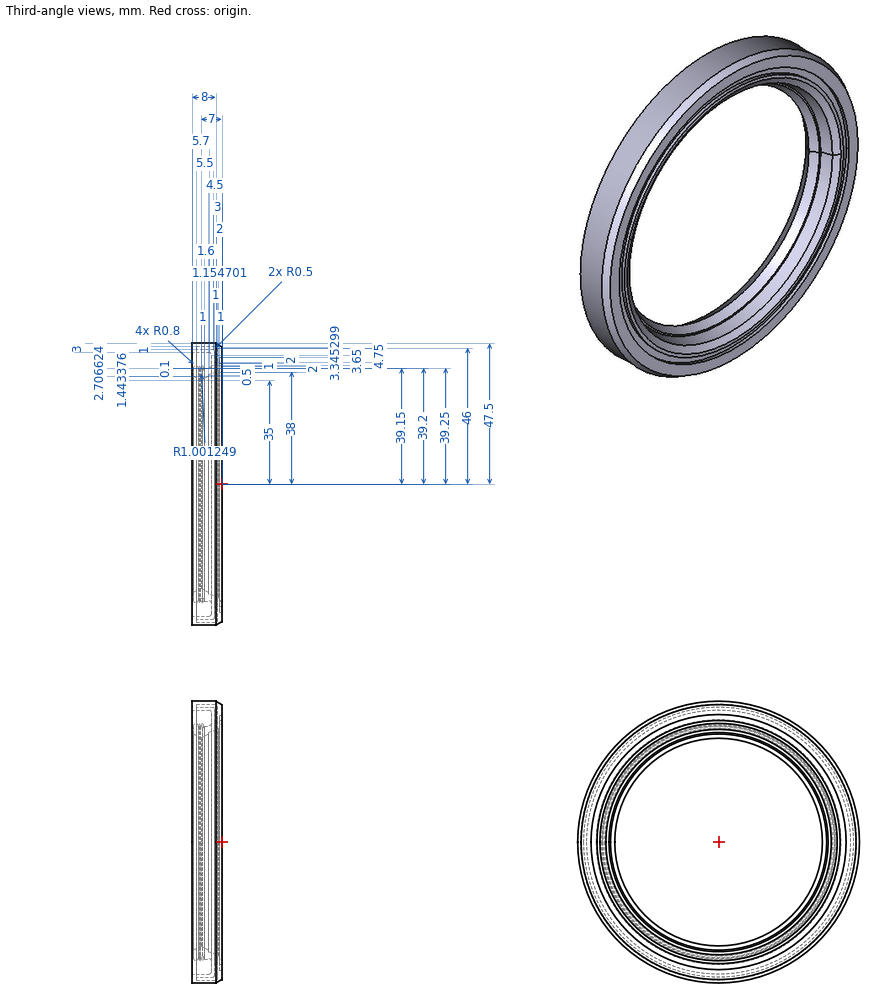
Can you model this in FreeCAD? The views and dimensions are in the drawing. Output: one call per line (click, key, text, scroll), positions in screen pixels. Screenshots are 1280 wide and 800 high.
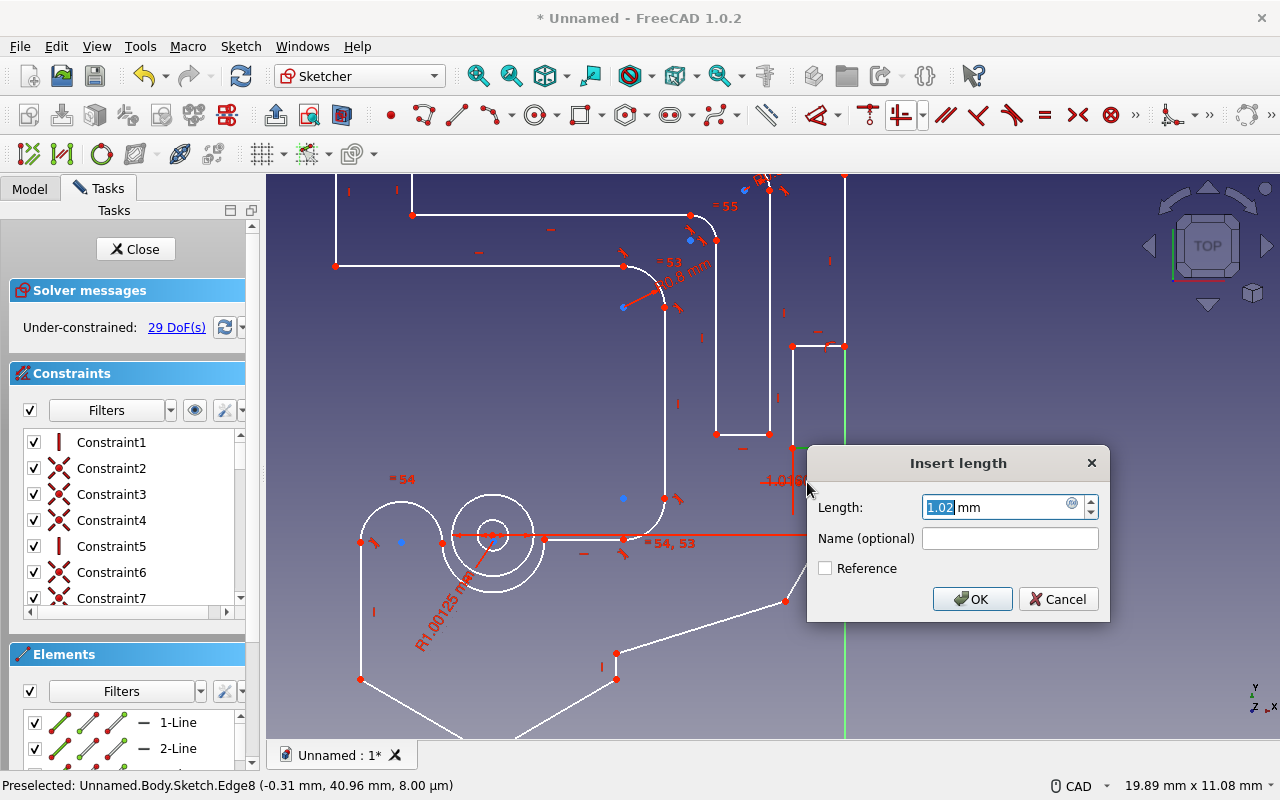
text(1)
key(Return)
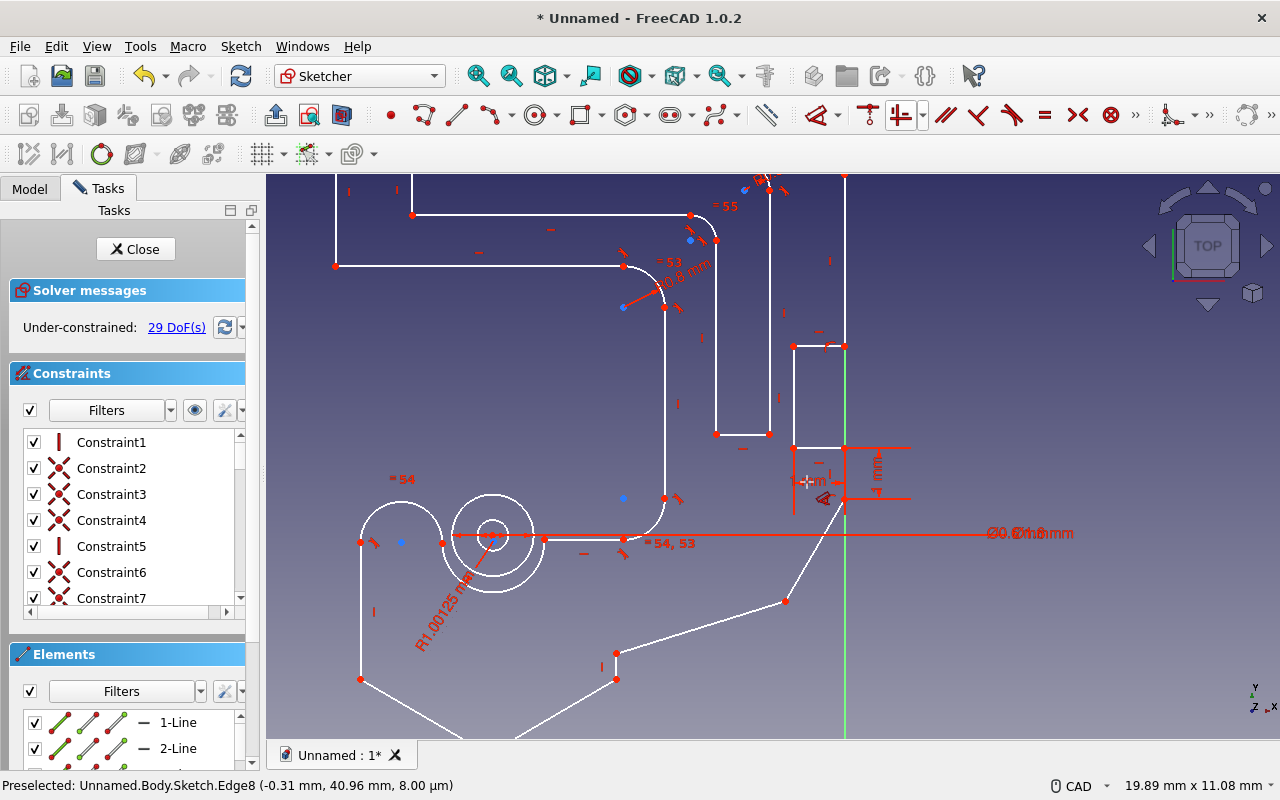
click(794, 417)
click(828, 397)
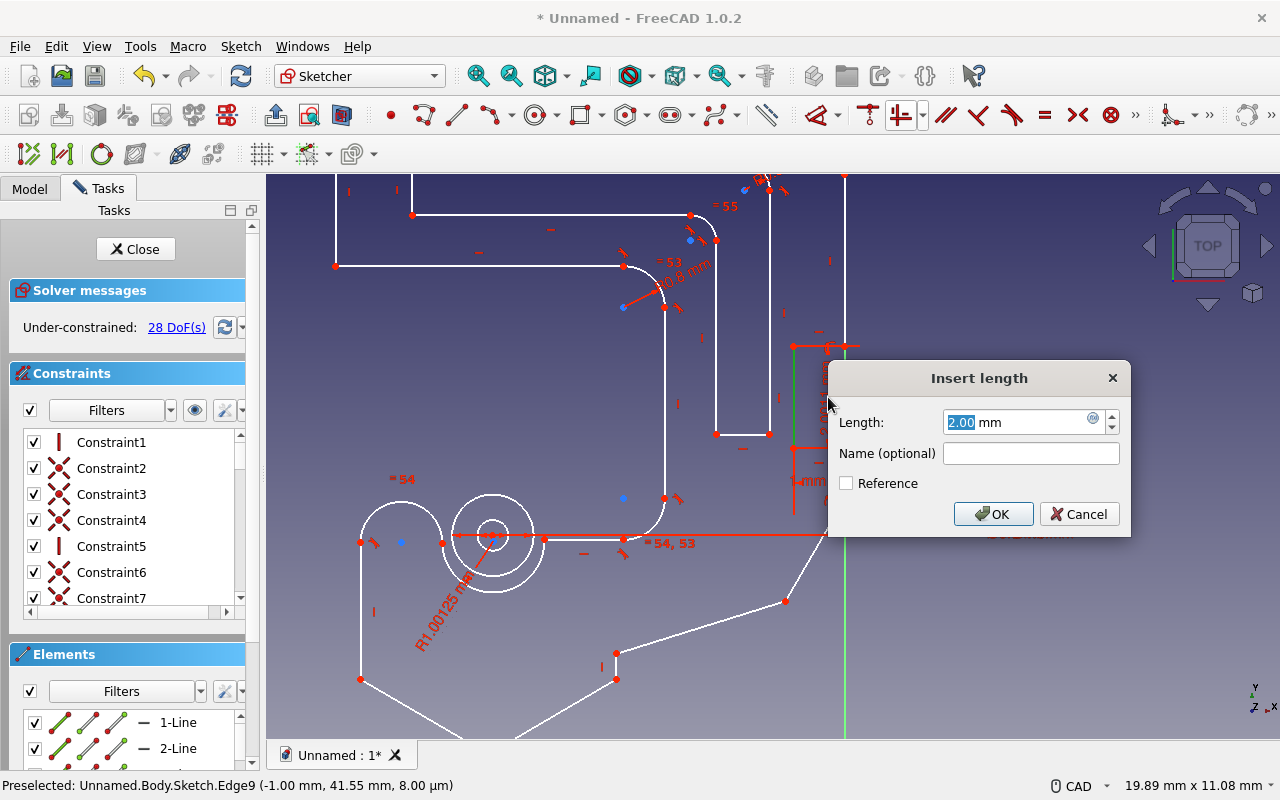
text(2)
key(Return)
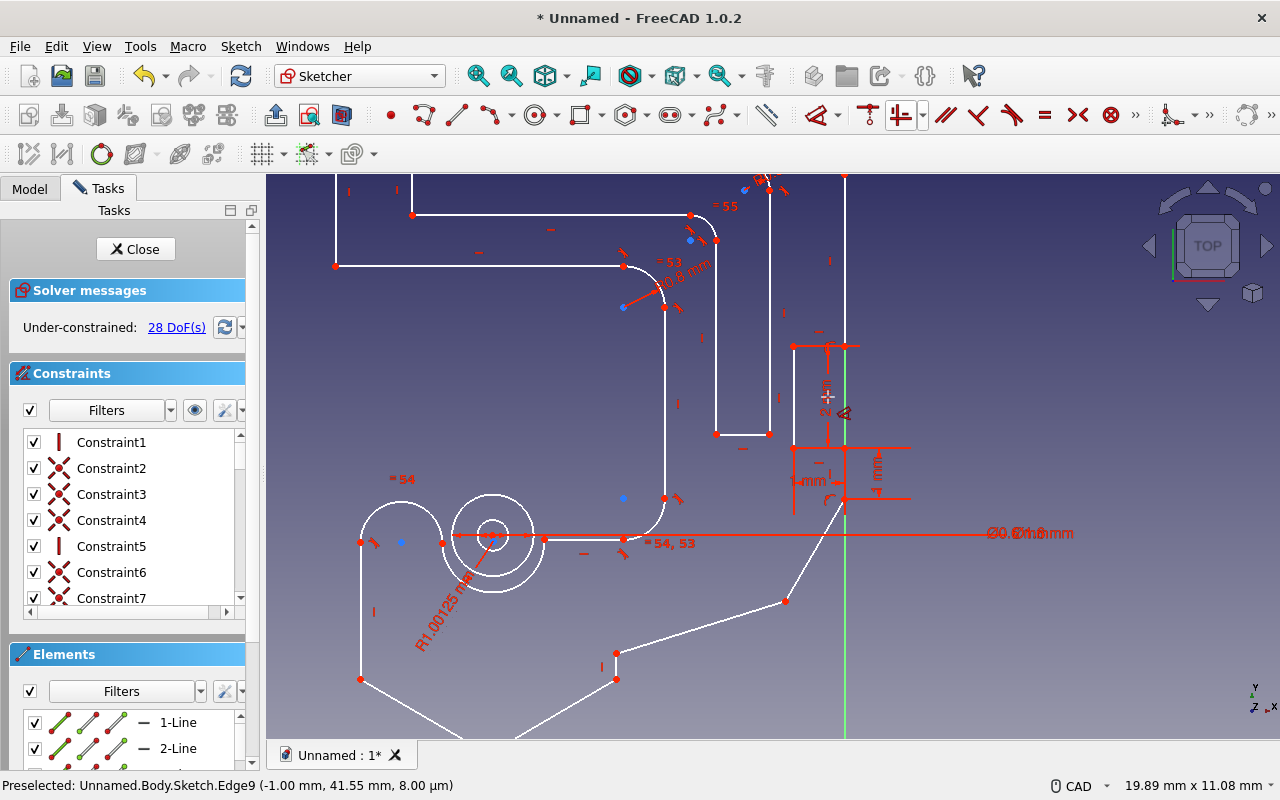
scroll(844, 485, down, 3)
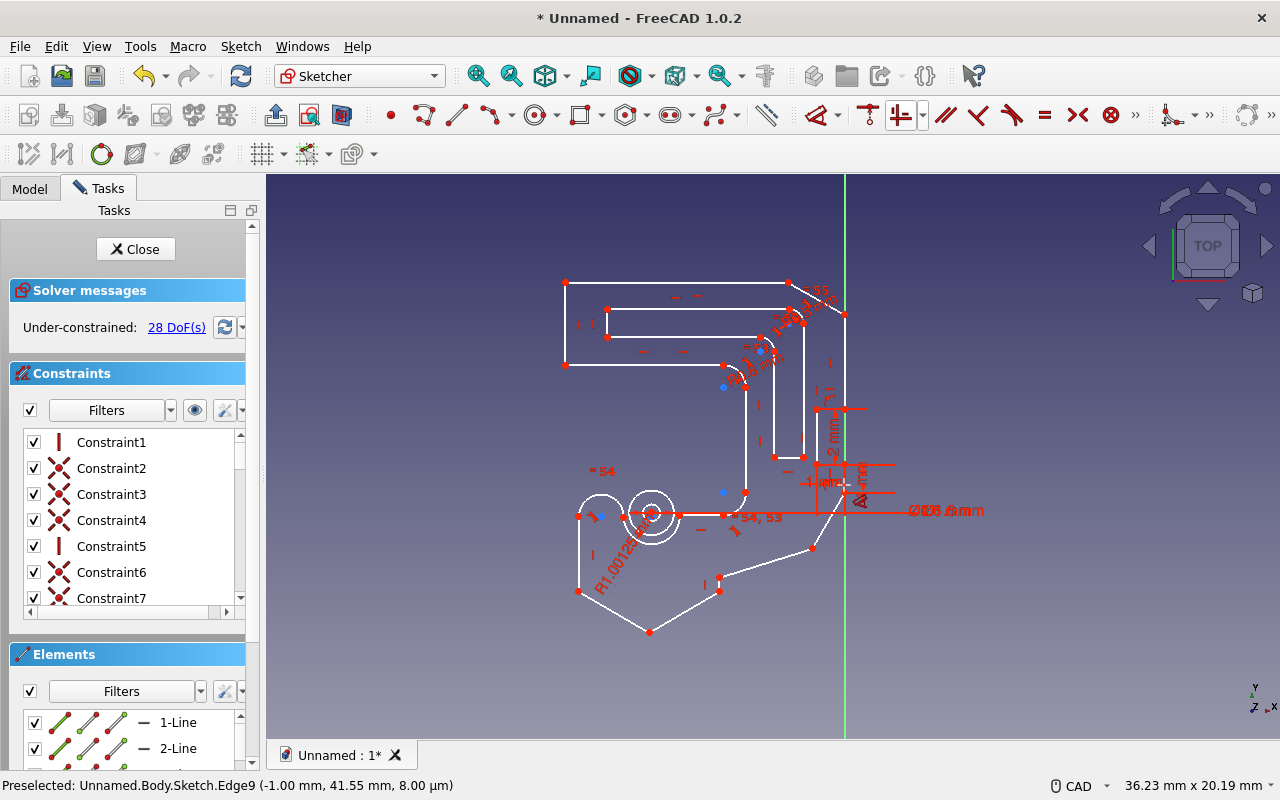
click(721, 283)
click(677, 249)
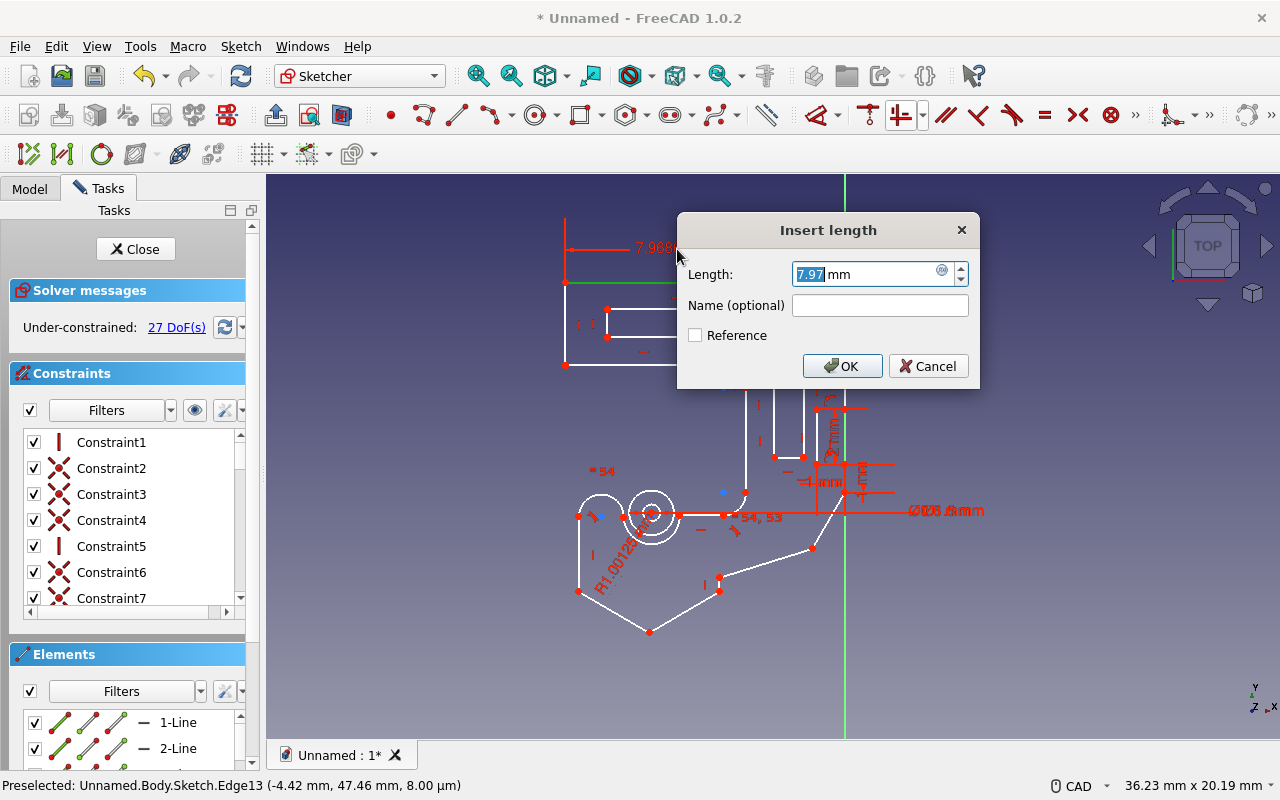
text(8)
key(Return)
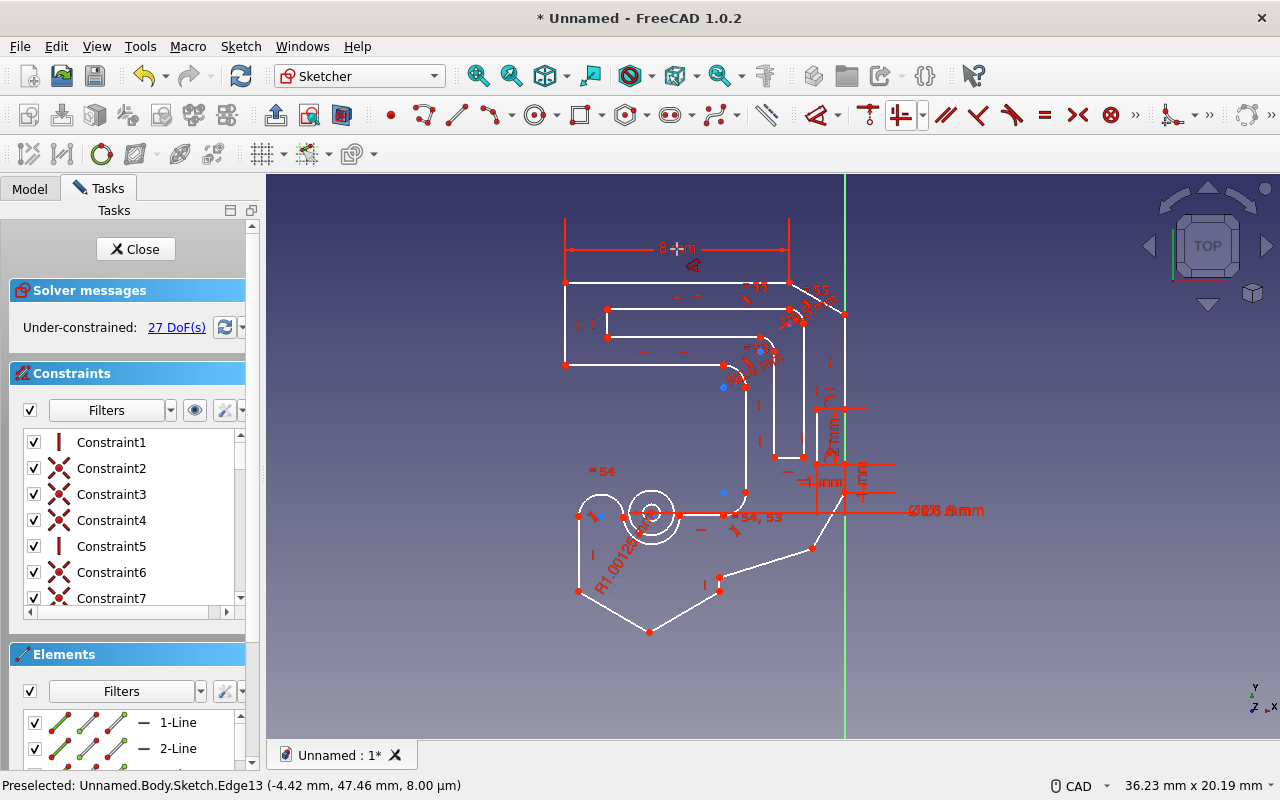
click(565, 308)
click(531, 324)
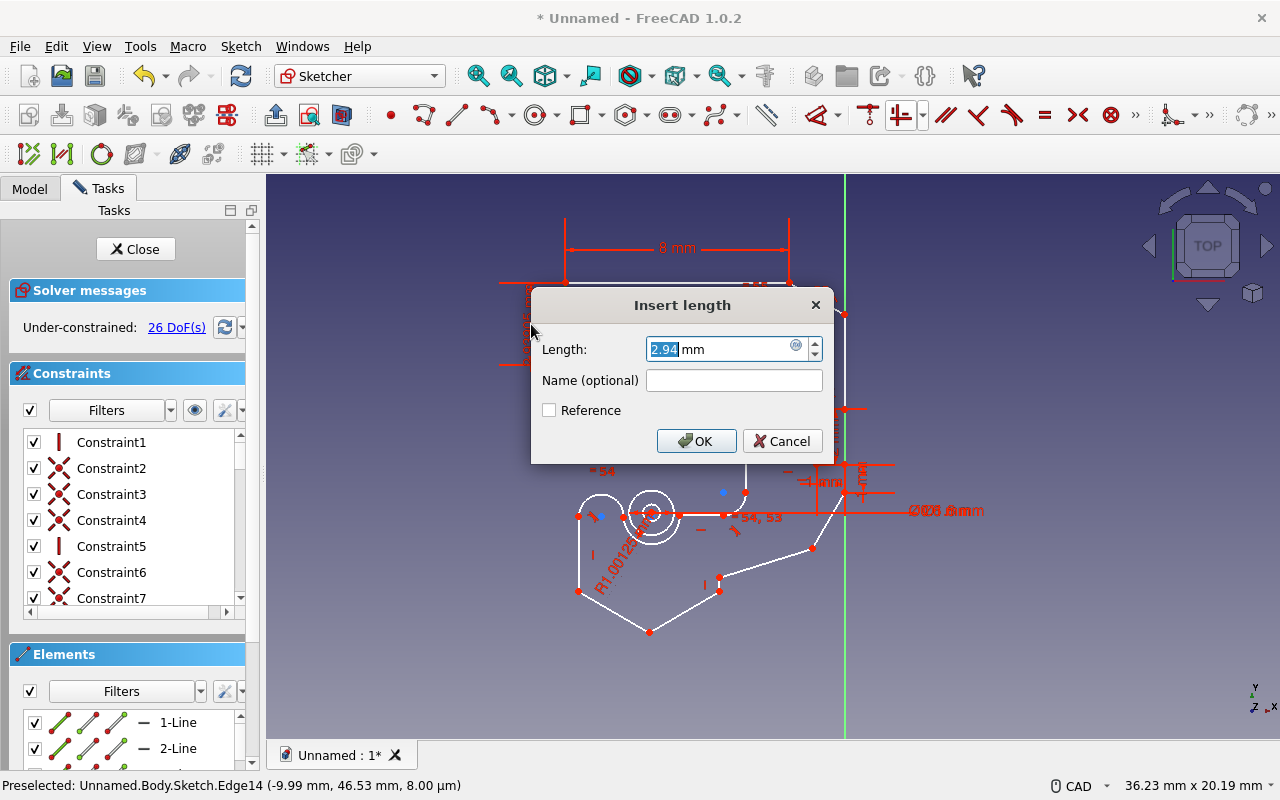
text(3)
key(Return)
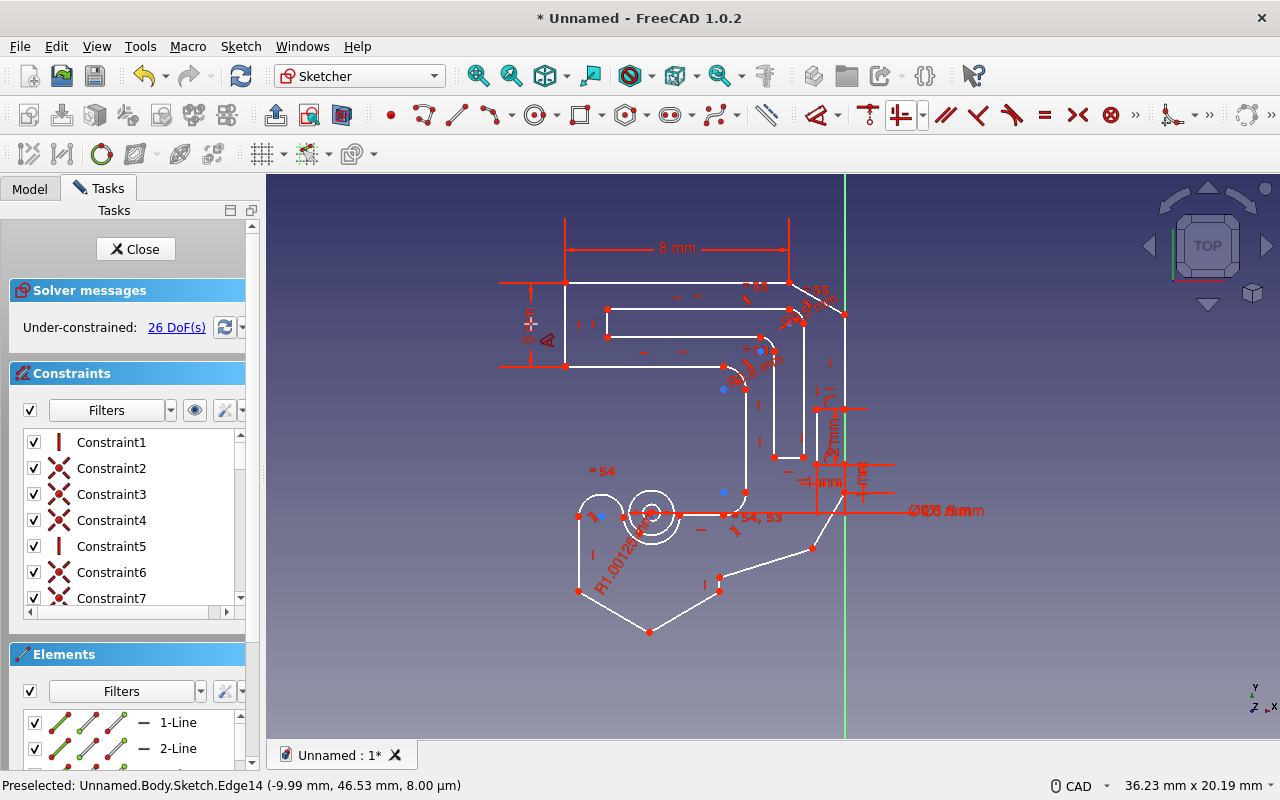
scroll(607, 326, up, 2)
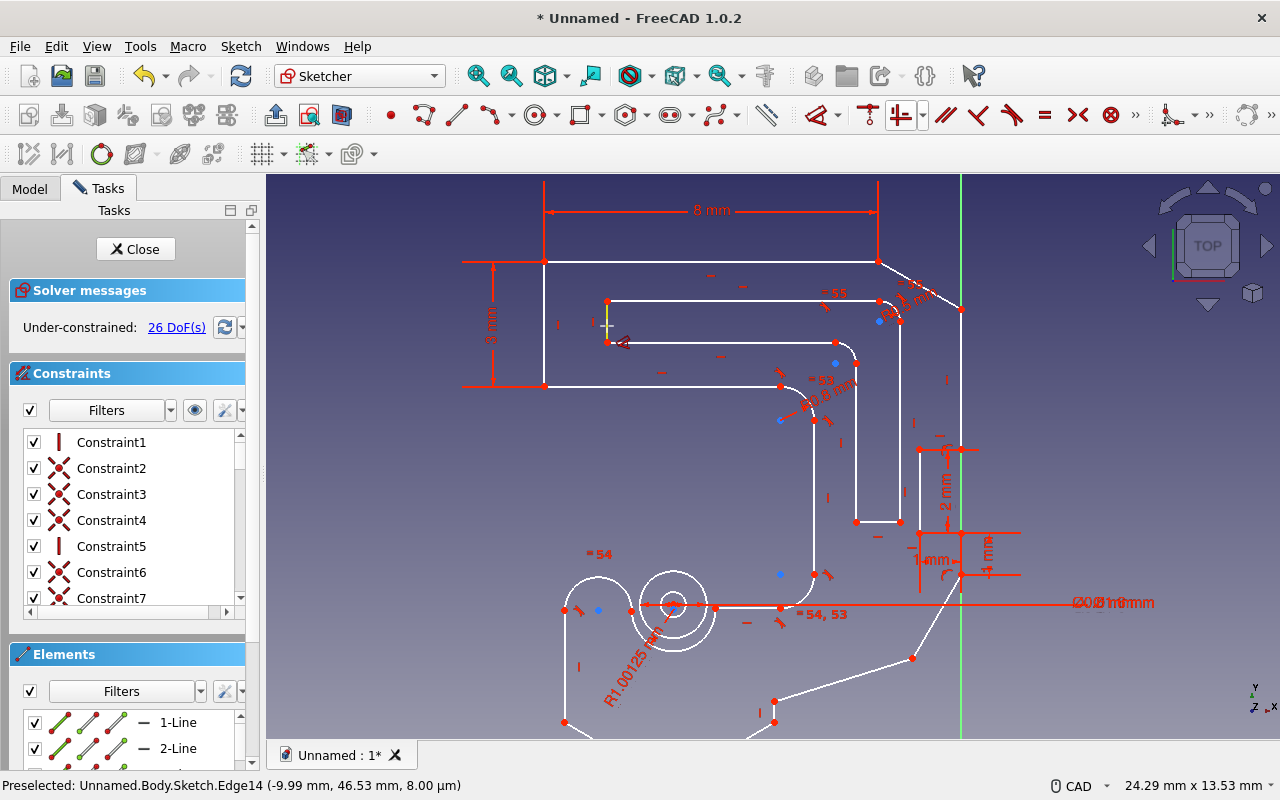
click(607, 326)
click(573, 322)